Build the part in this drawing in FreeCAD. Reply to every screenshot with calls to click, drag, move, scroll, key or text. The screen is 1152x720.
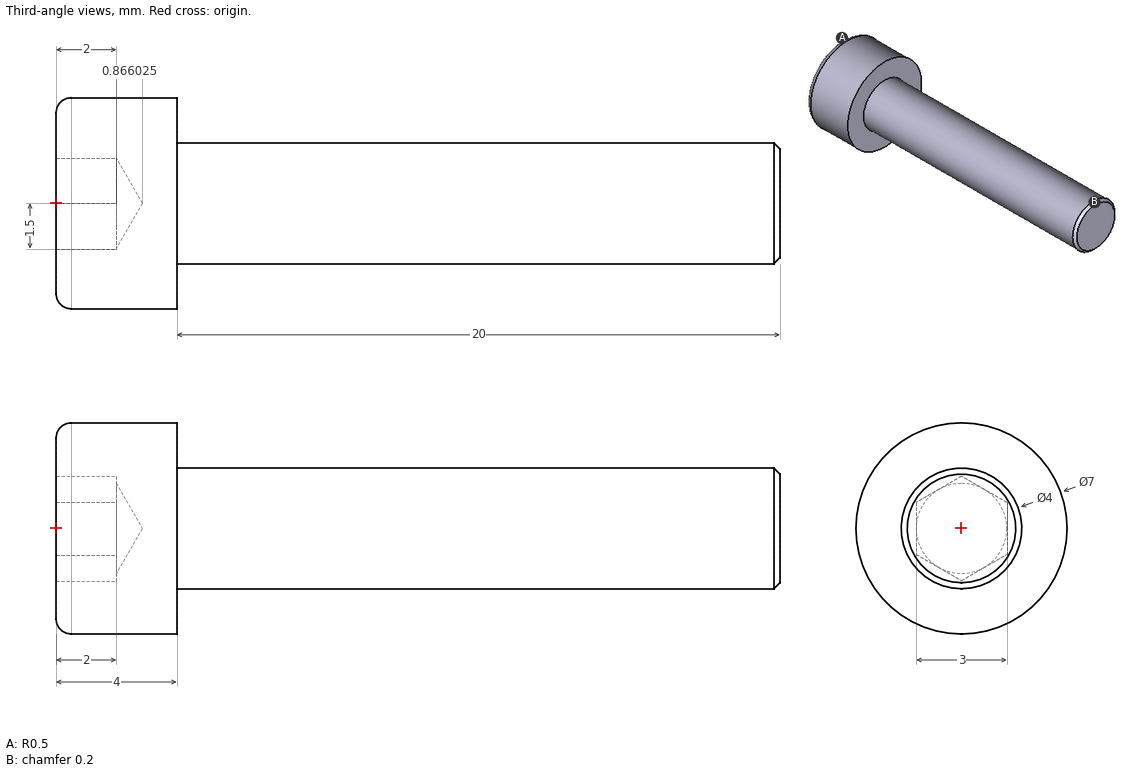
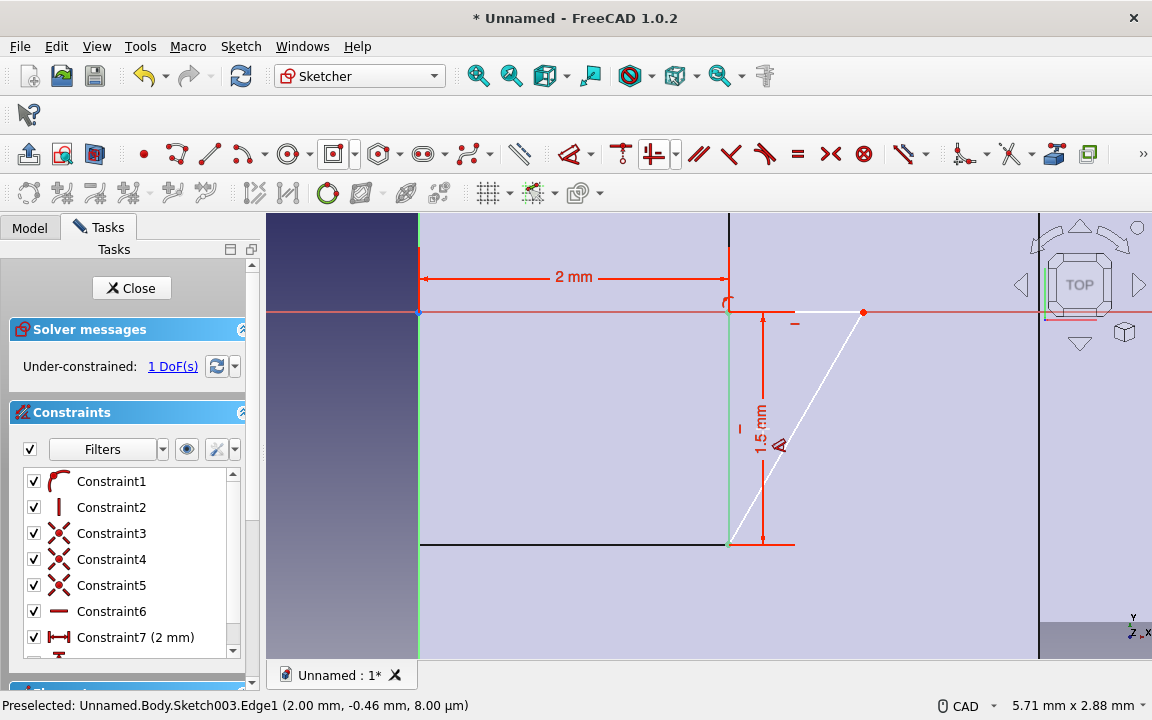
click(823, 312)
click(796, 278)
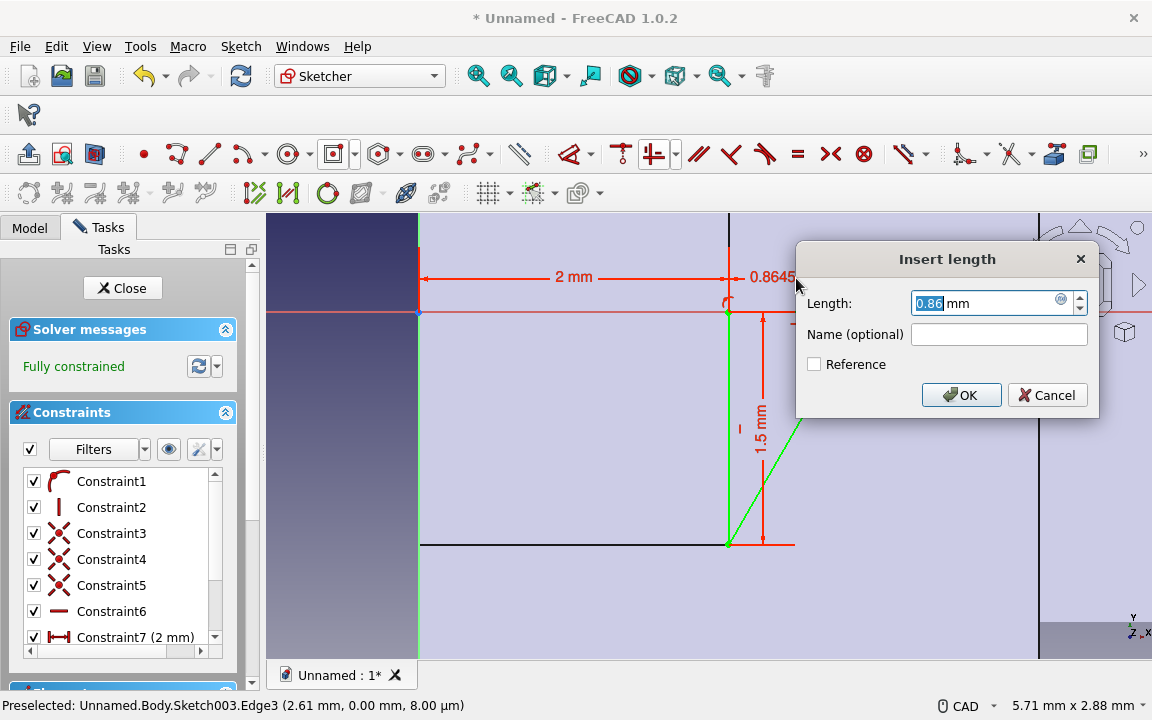
text(0.866025)
key(Return)
key(Escape)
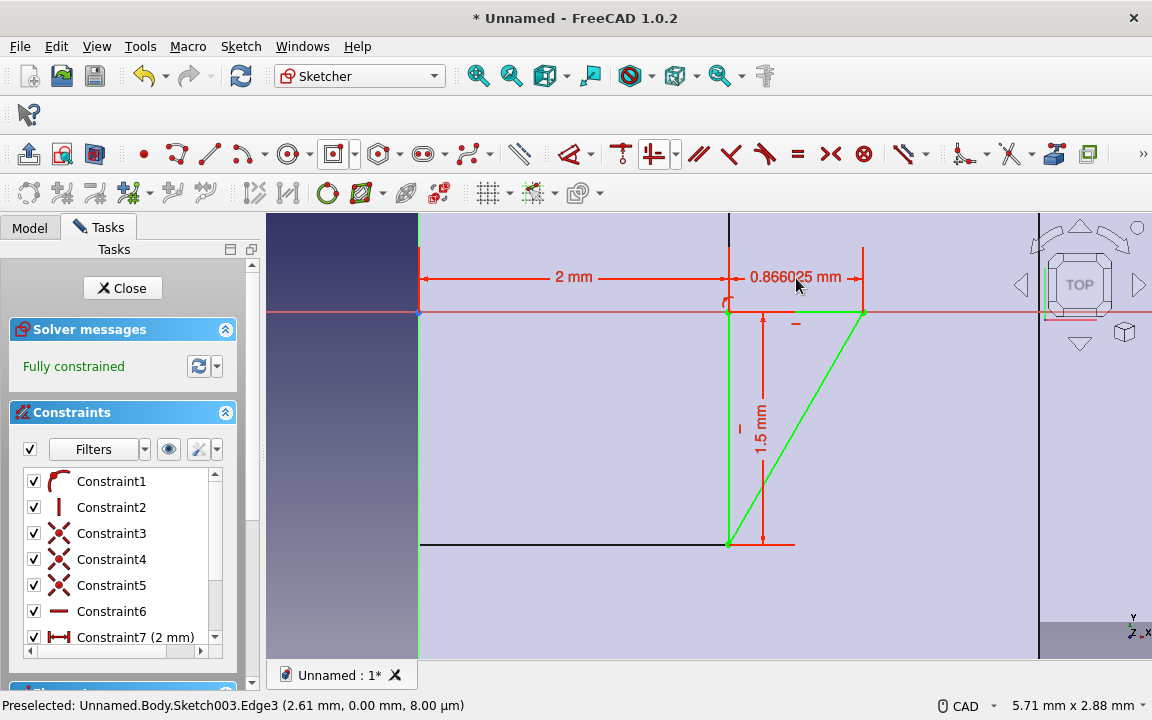
click(123, 288)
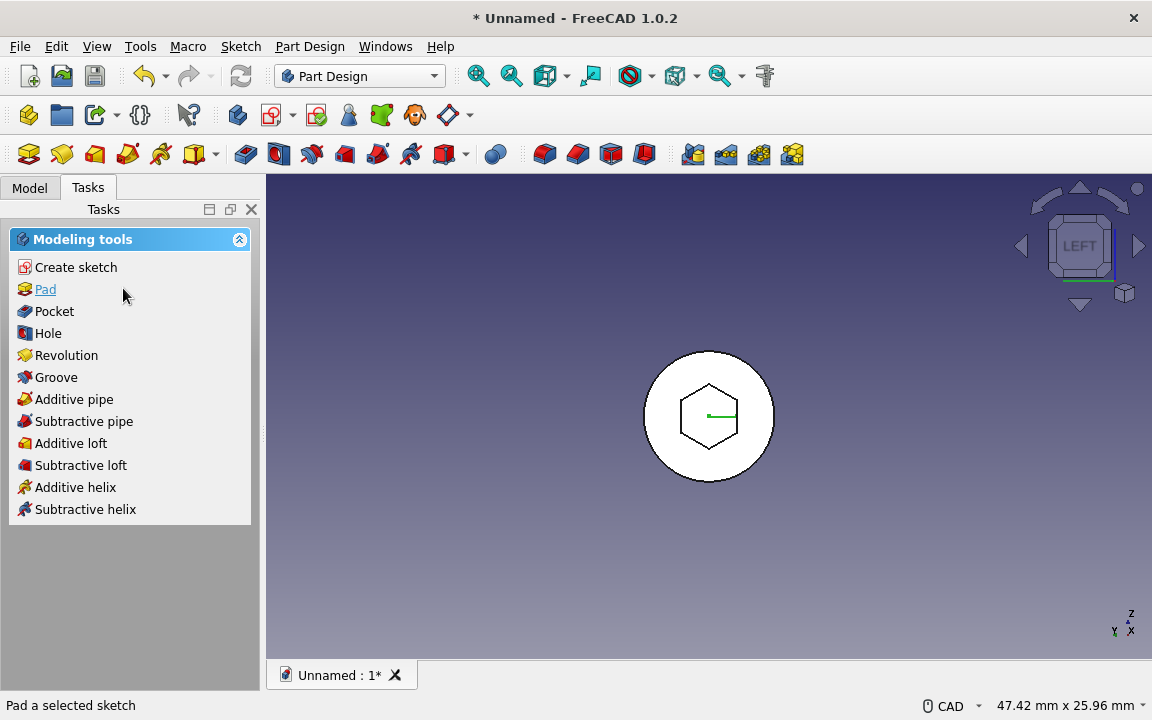
click(312, 154)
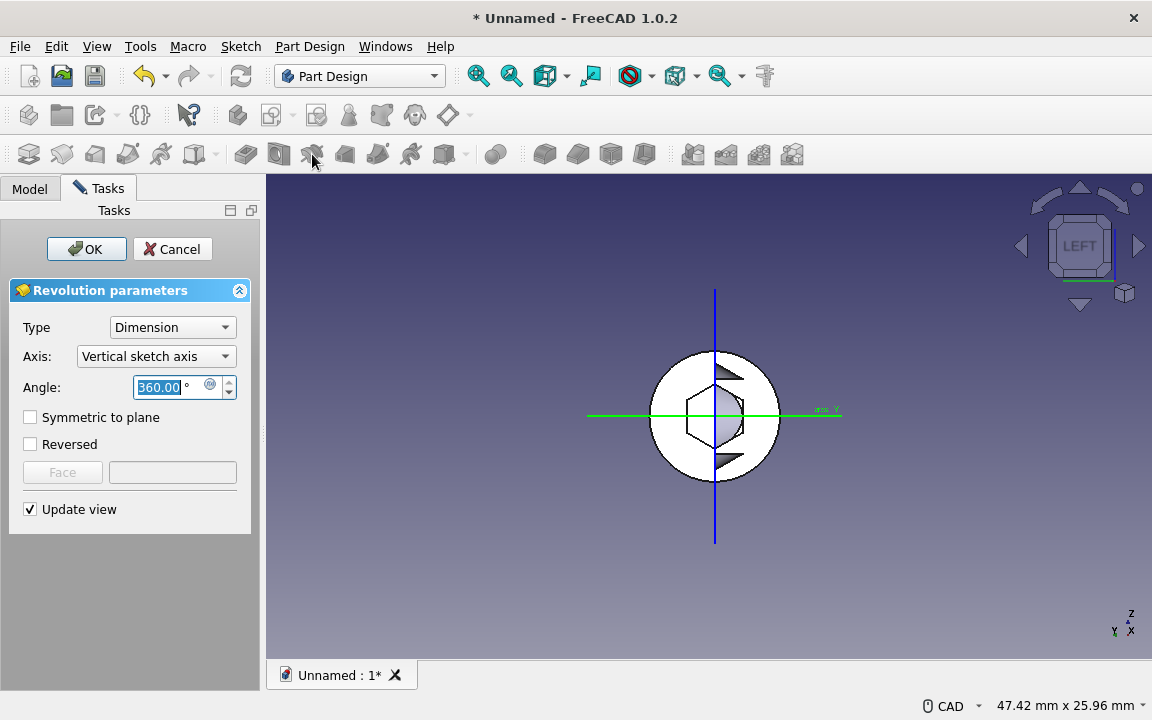
click(157, 356)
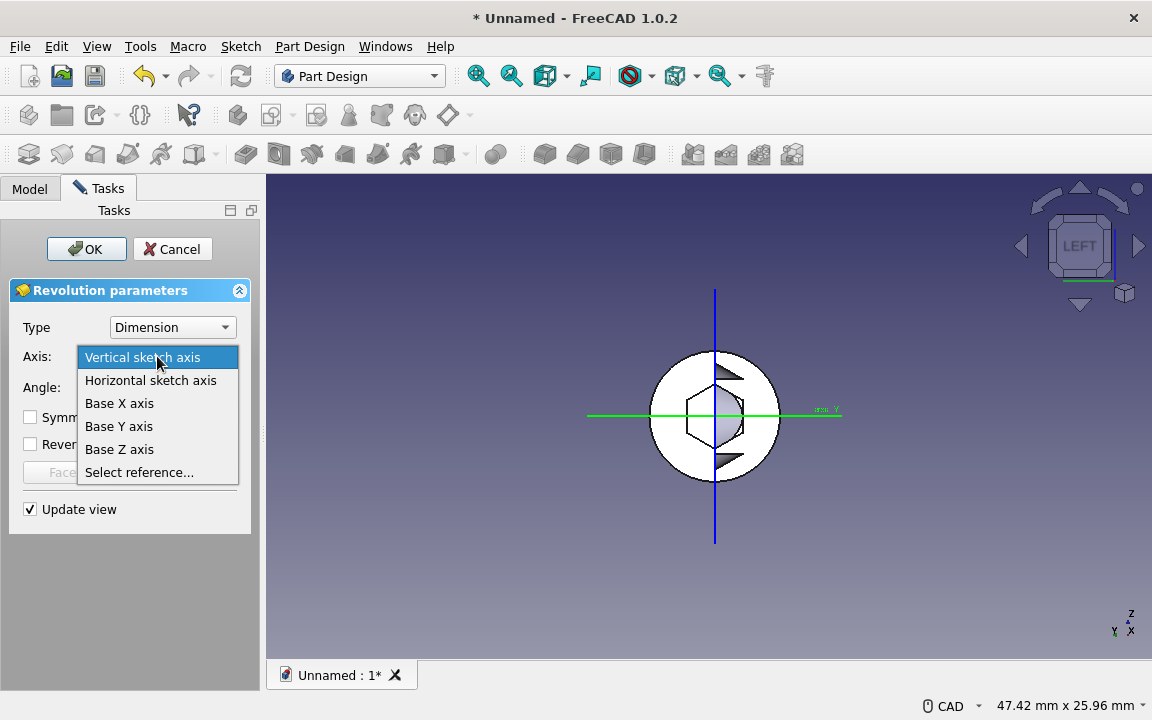
click(156, 380)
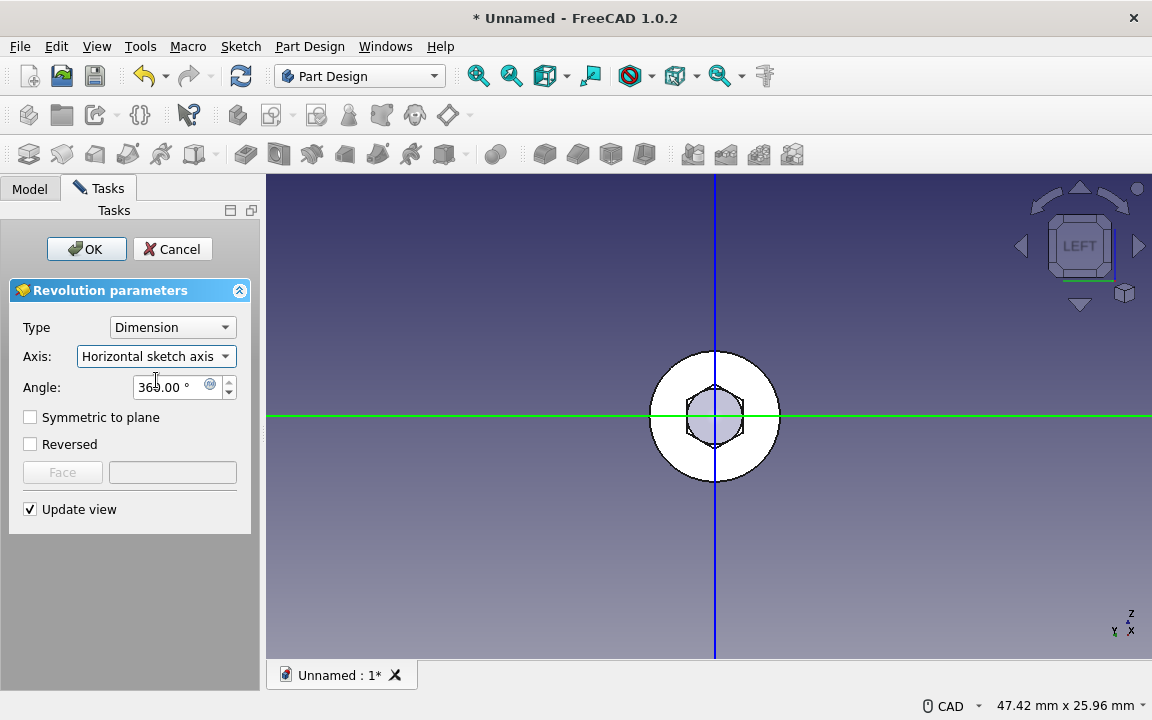
click(87, 249)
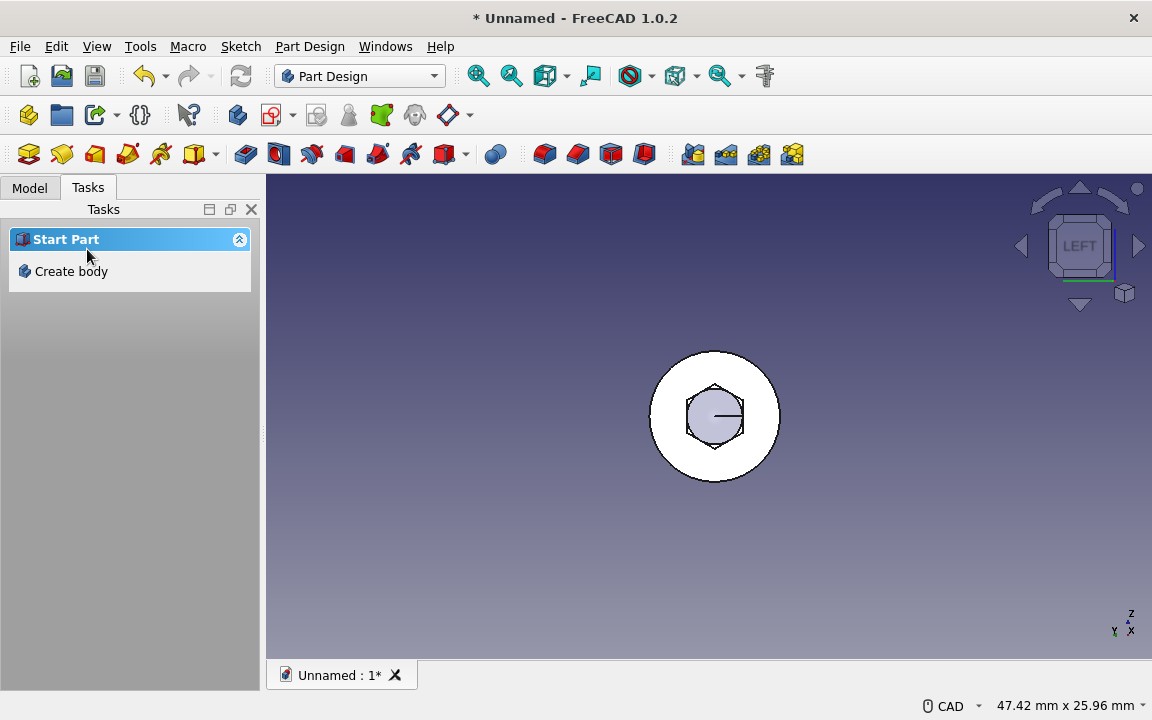
click(479, 76)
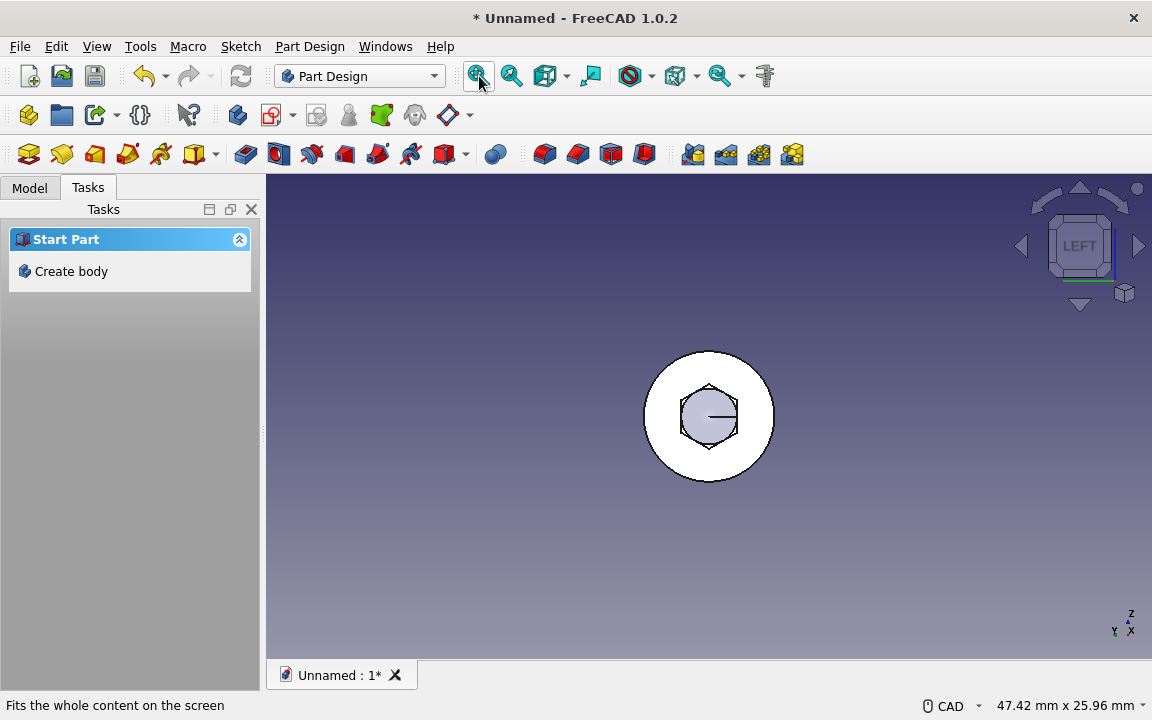
click(762, 377)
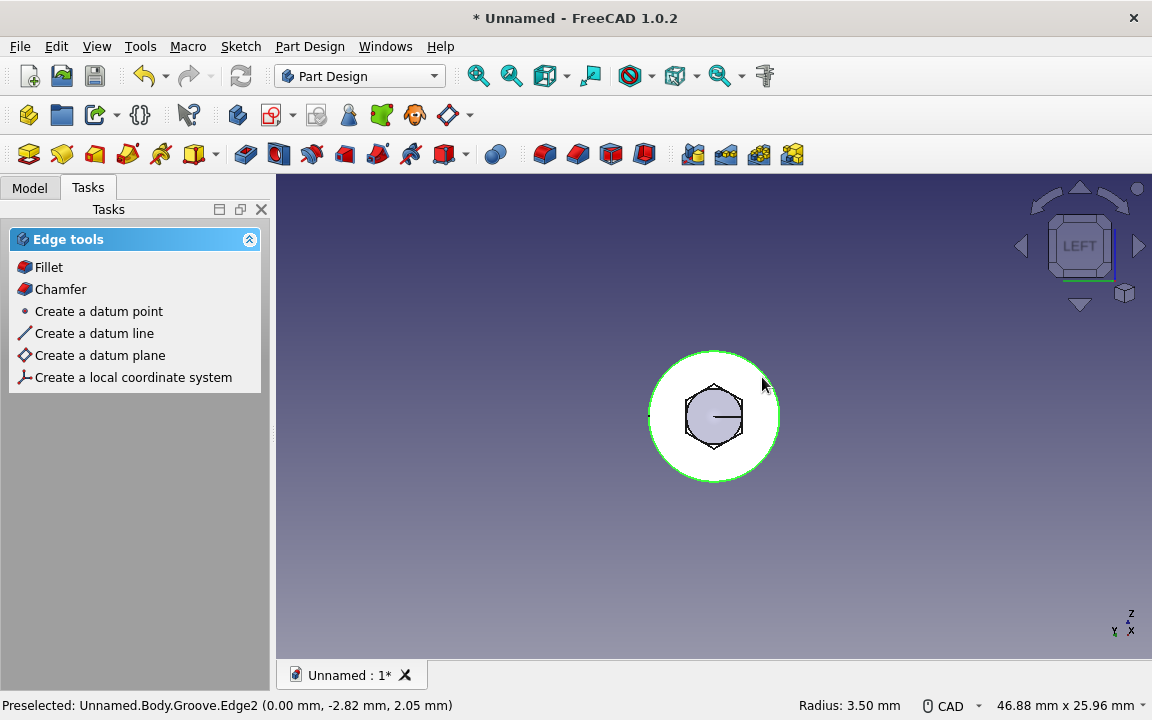
click(545, 154)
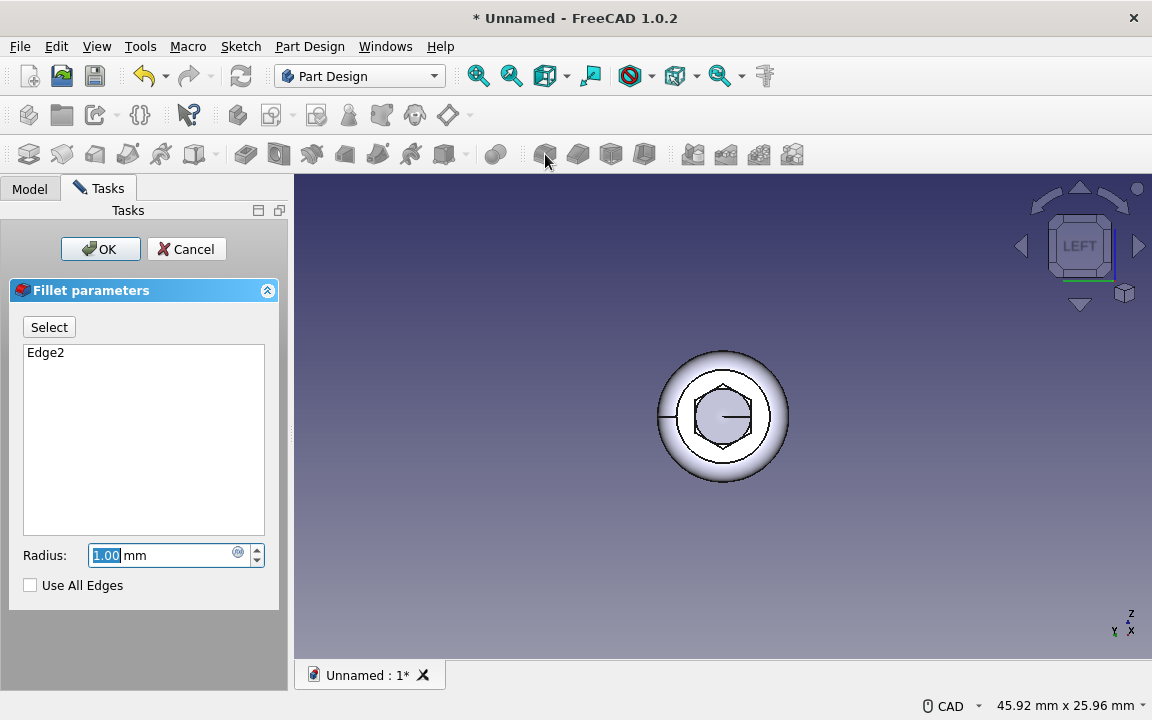
text(0.5)
key(Tab)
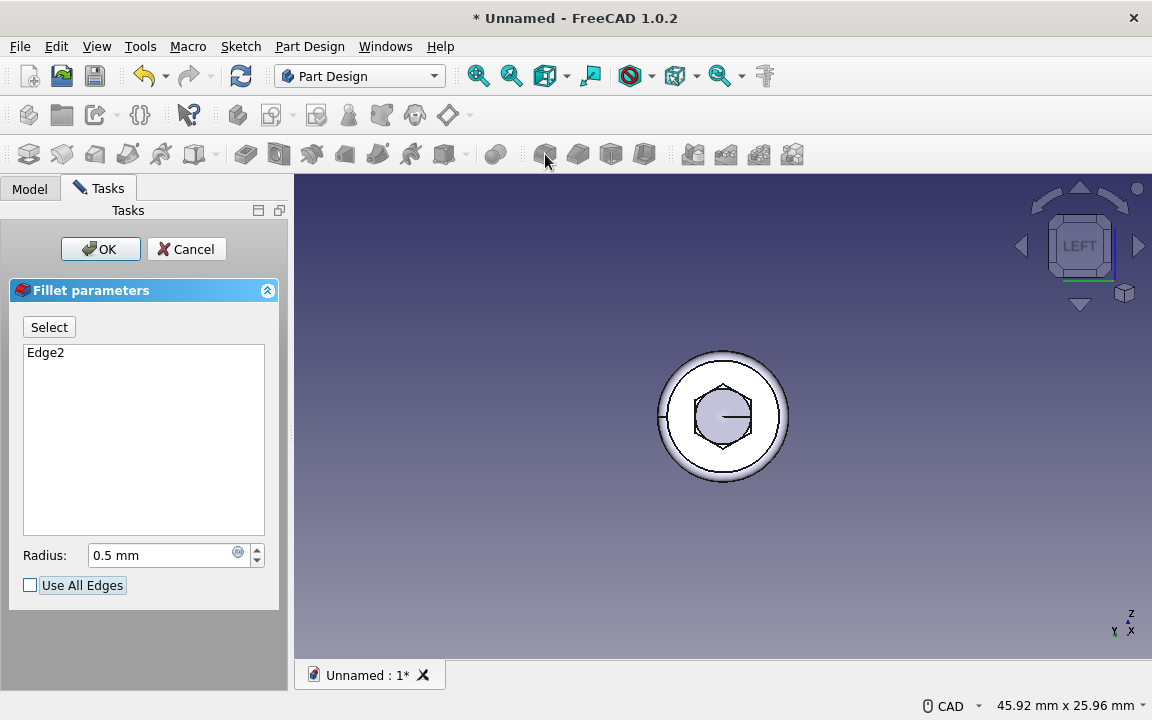
click(101, 249)